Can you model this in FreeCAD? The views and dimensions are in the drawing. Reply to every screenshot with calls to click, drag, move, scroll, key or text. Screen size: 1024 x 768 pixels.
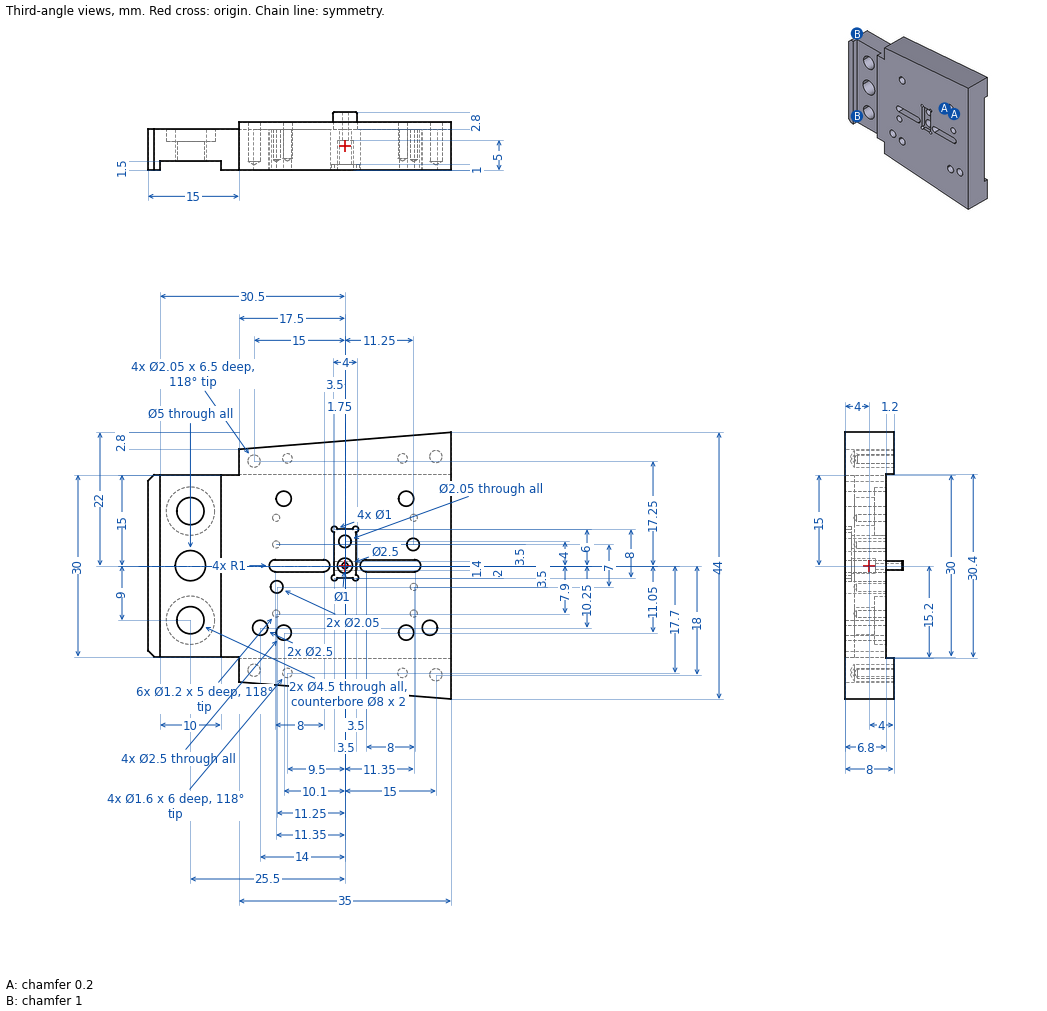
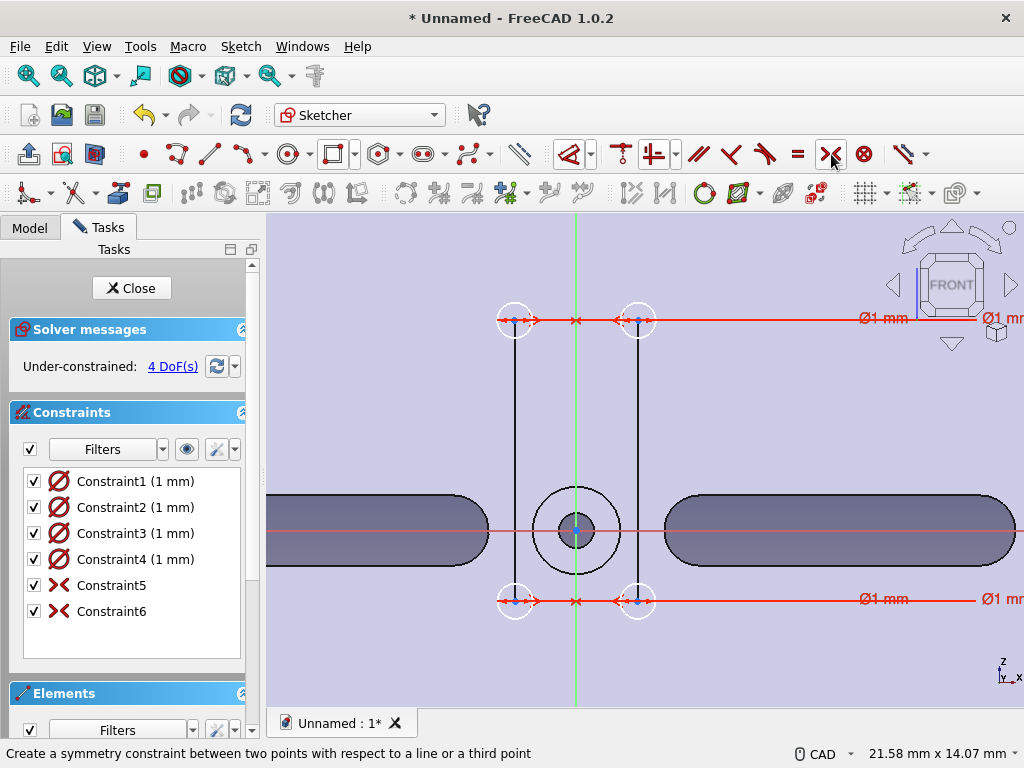
click(515, 320)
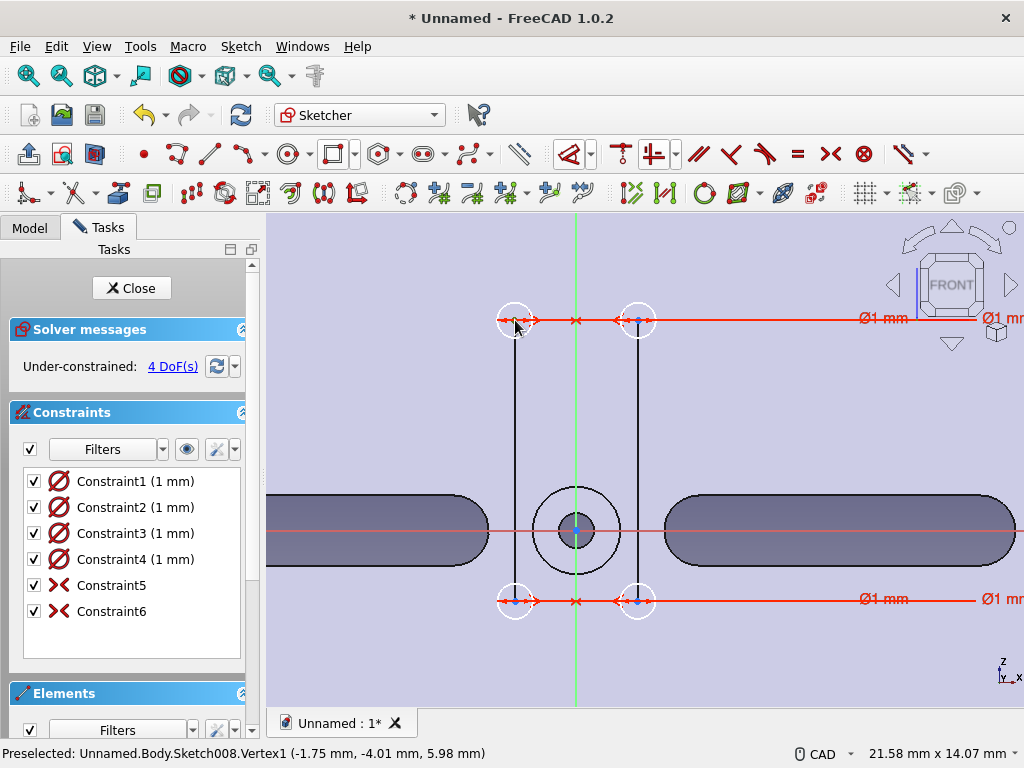
click(590, 154)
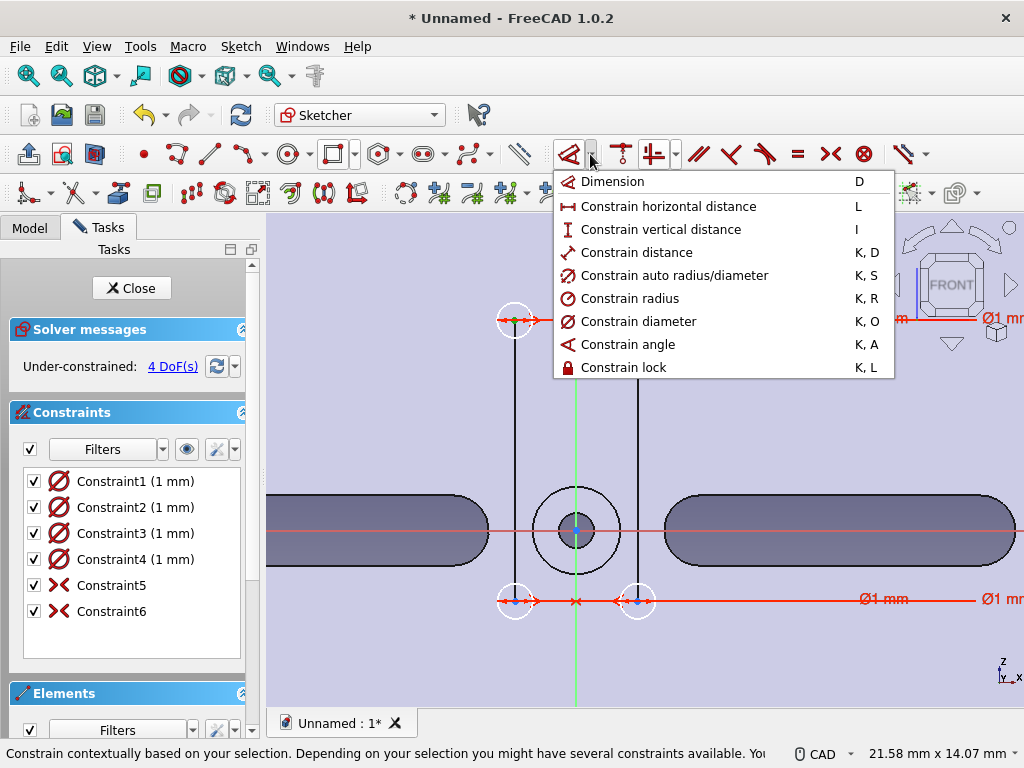
click(724, 230)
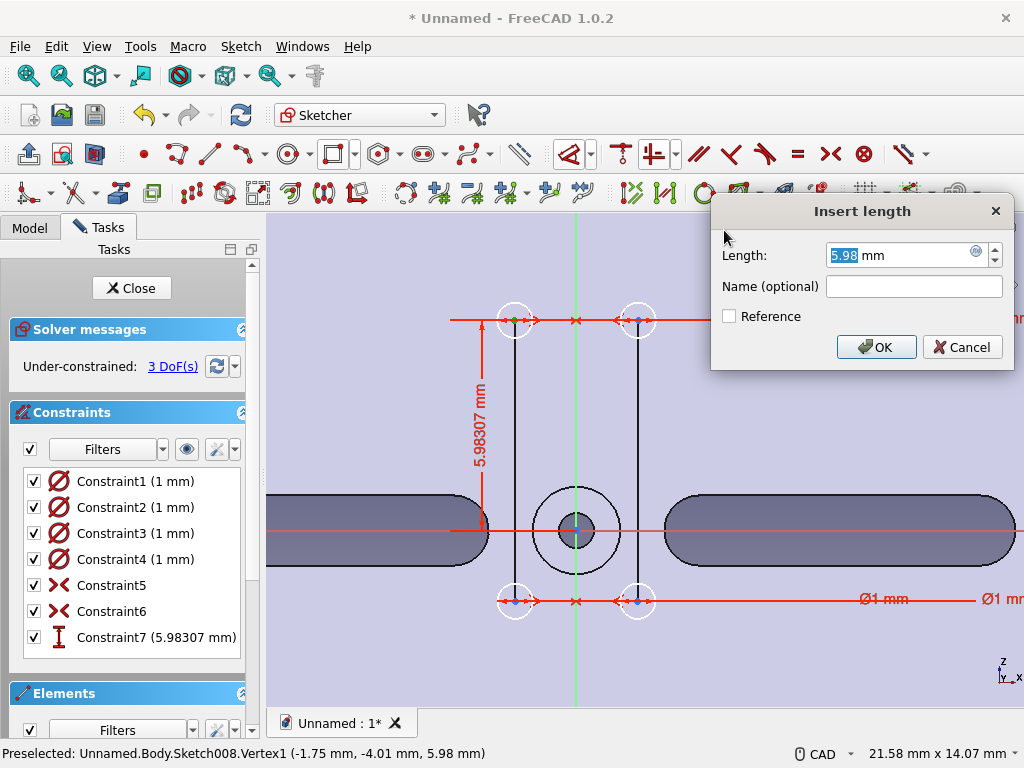
text(6)
key(Return)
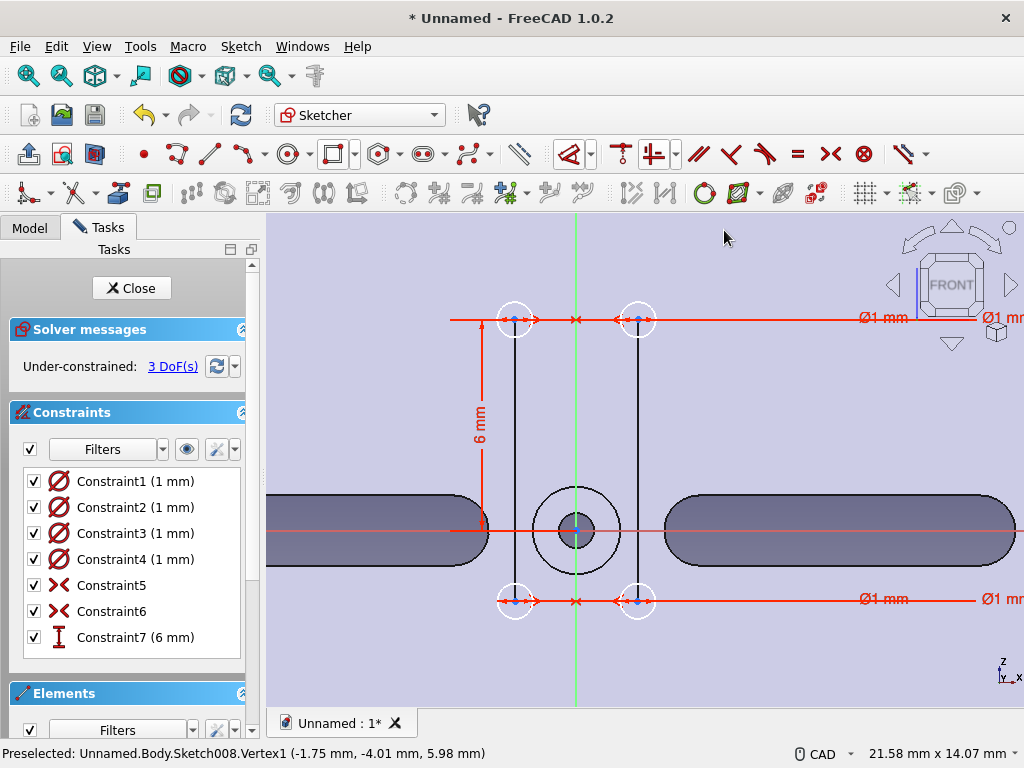
click(515, 601)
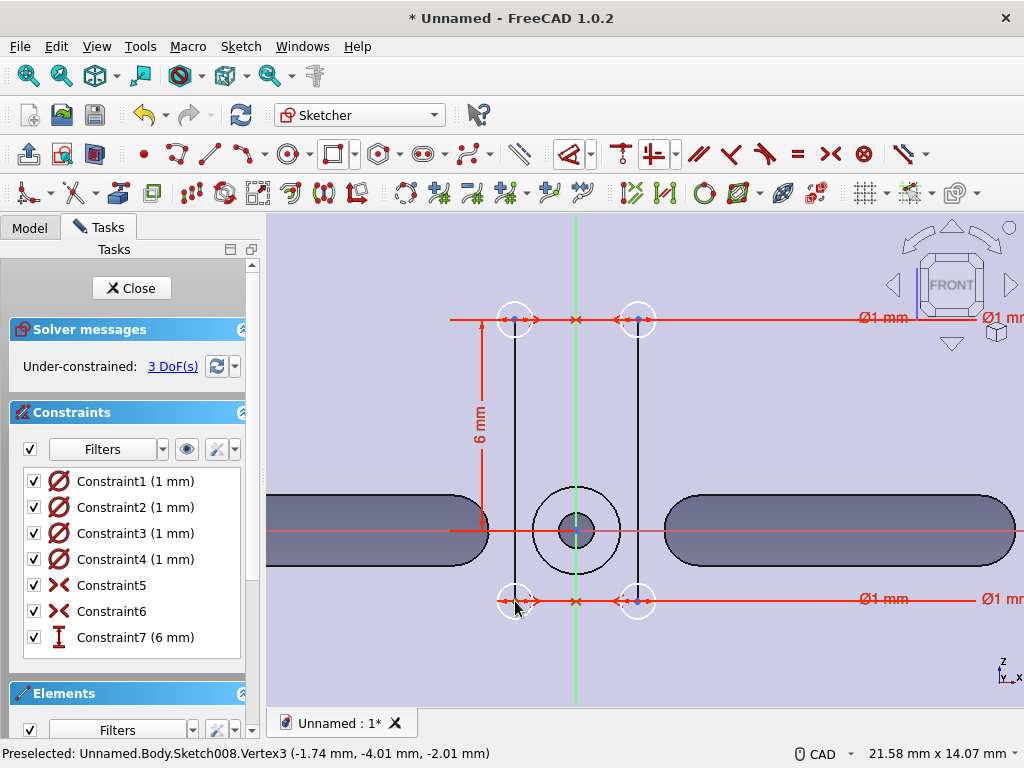
click(590, 154)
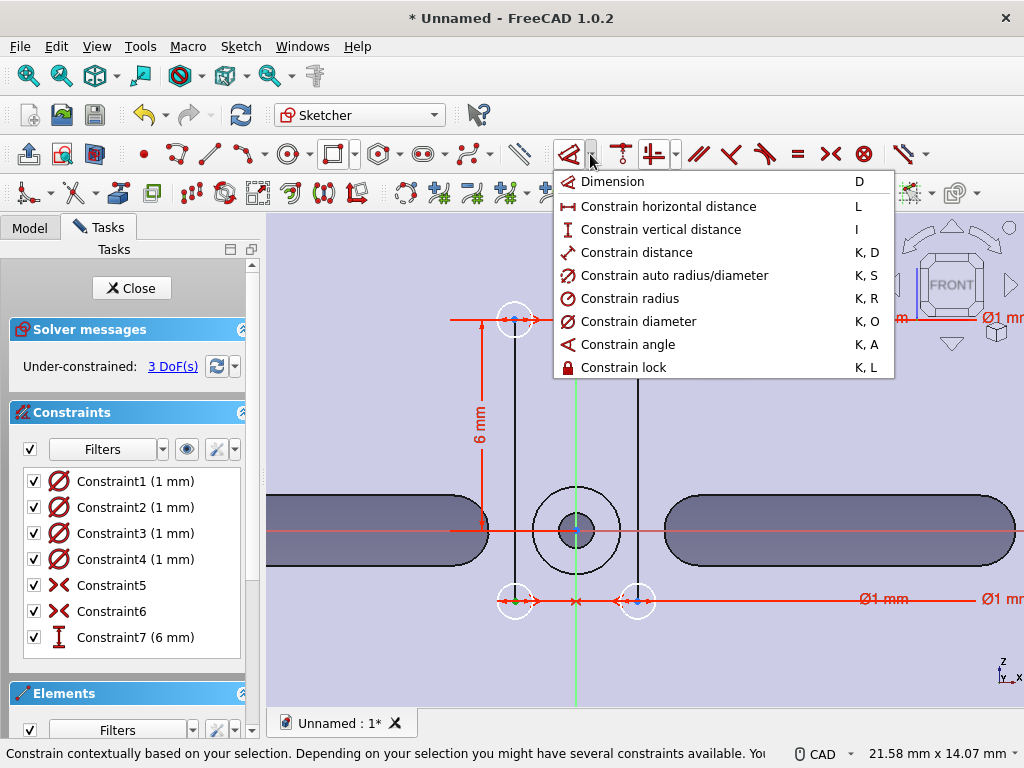
click(724, 230)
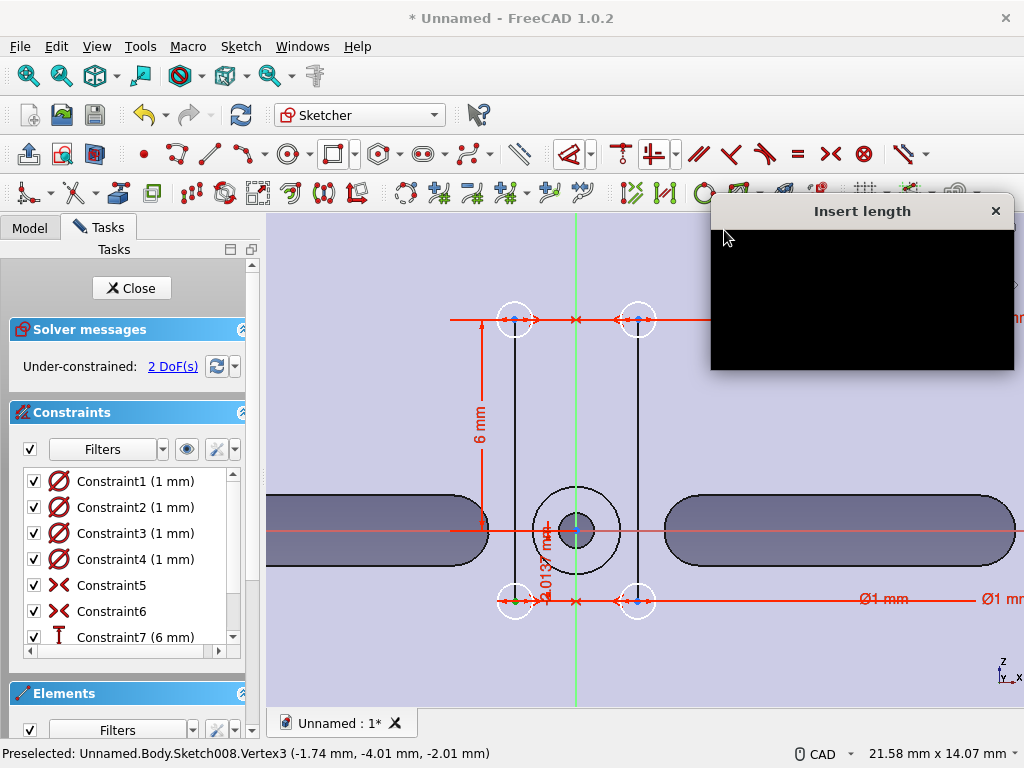
text(-2)
key(Return)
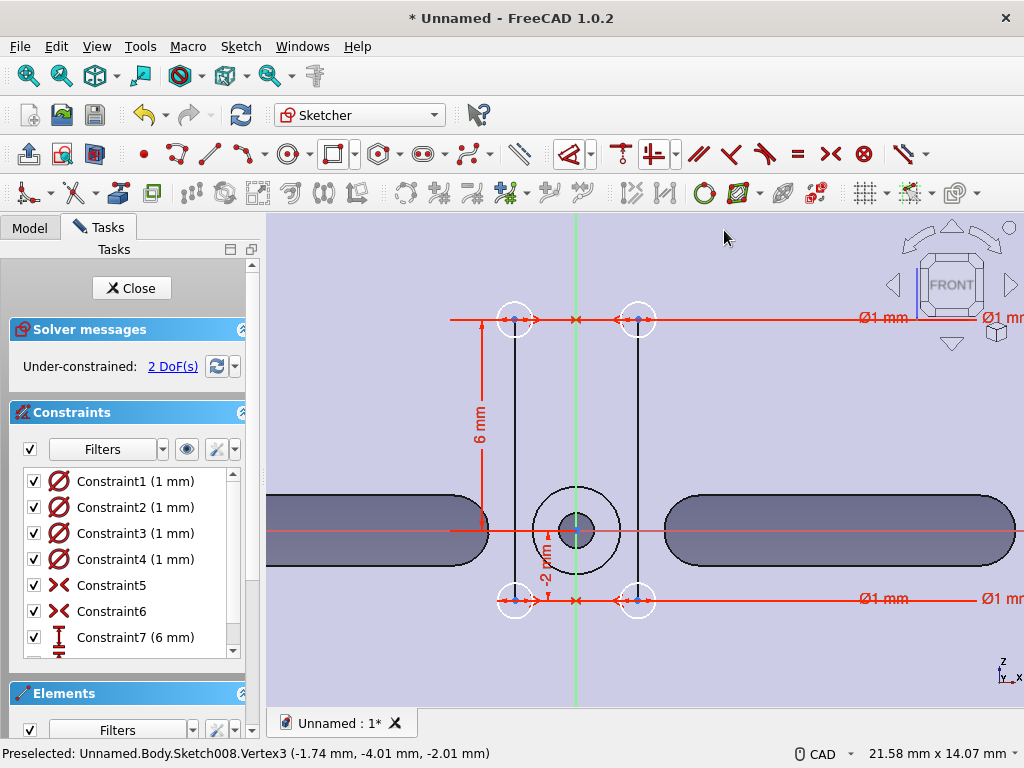
click(515, 320)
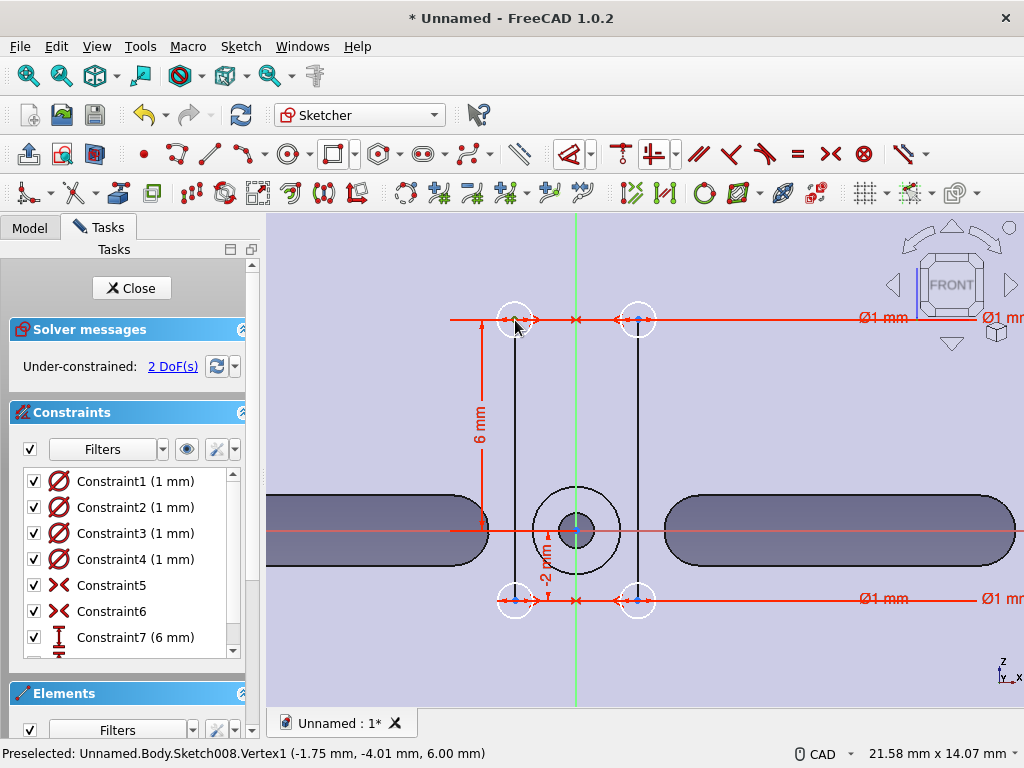
click(590, 154)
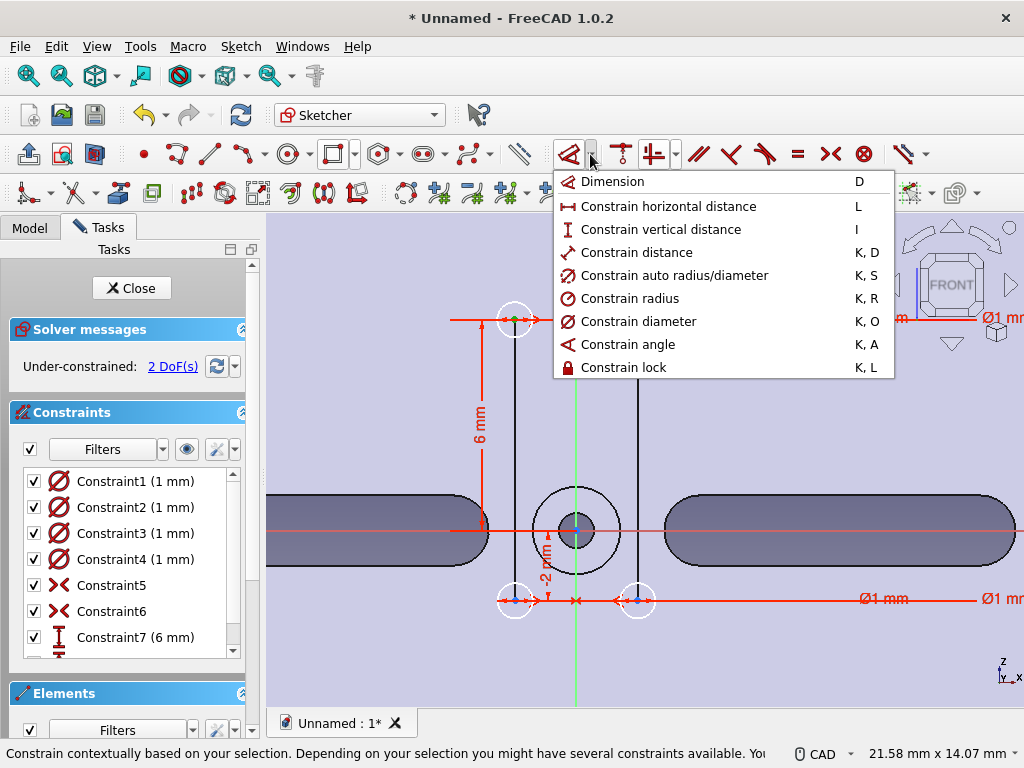
click(724, 206)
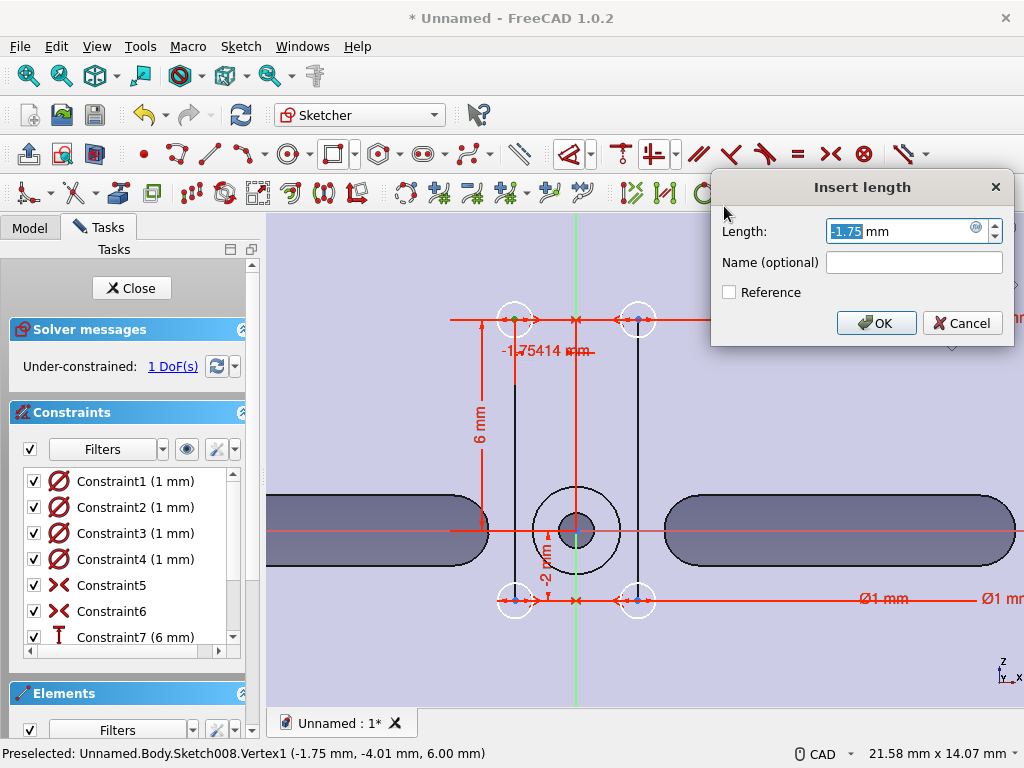
text(-1.75)
key(Return)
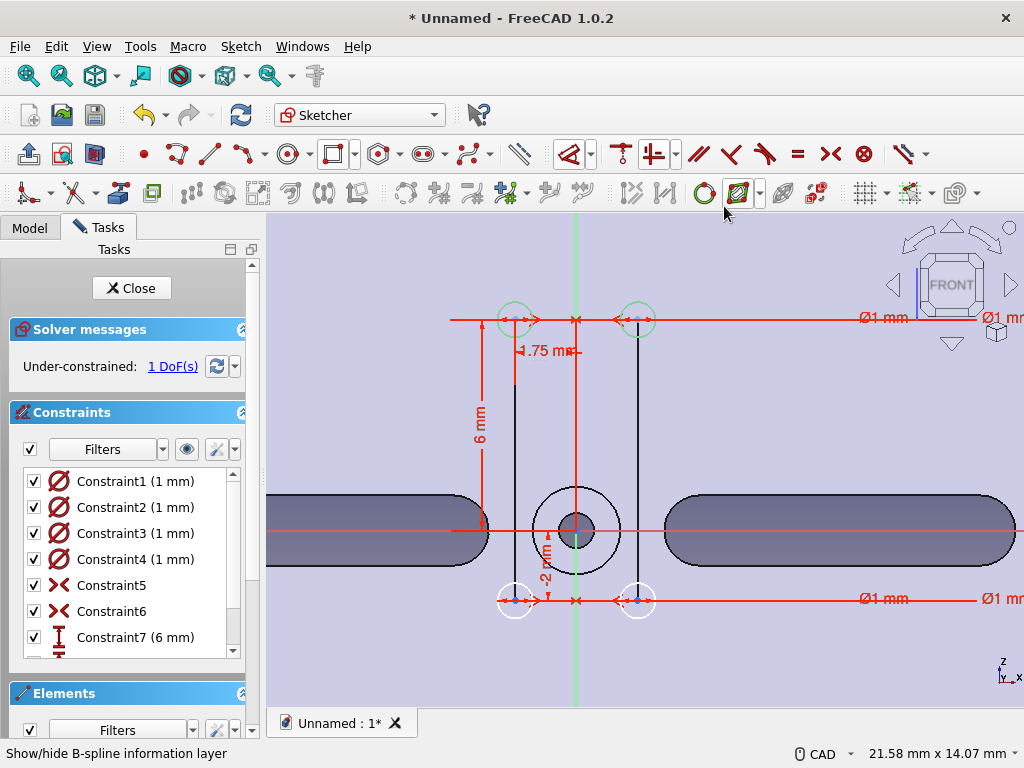
click(515, 601)